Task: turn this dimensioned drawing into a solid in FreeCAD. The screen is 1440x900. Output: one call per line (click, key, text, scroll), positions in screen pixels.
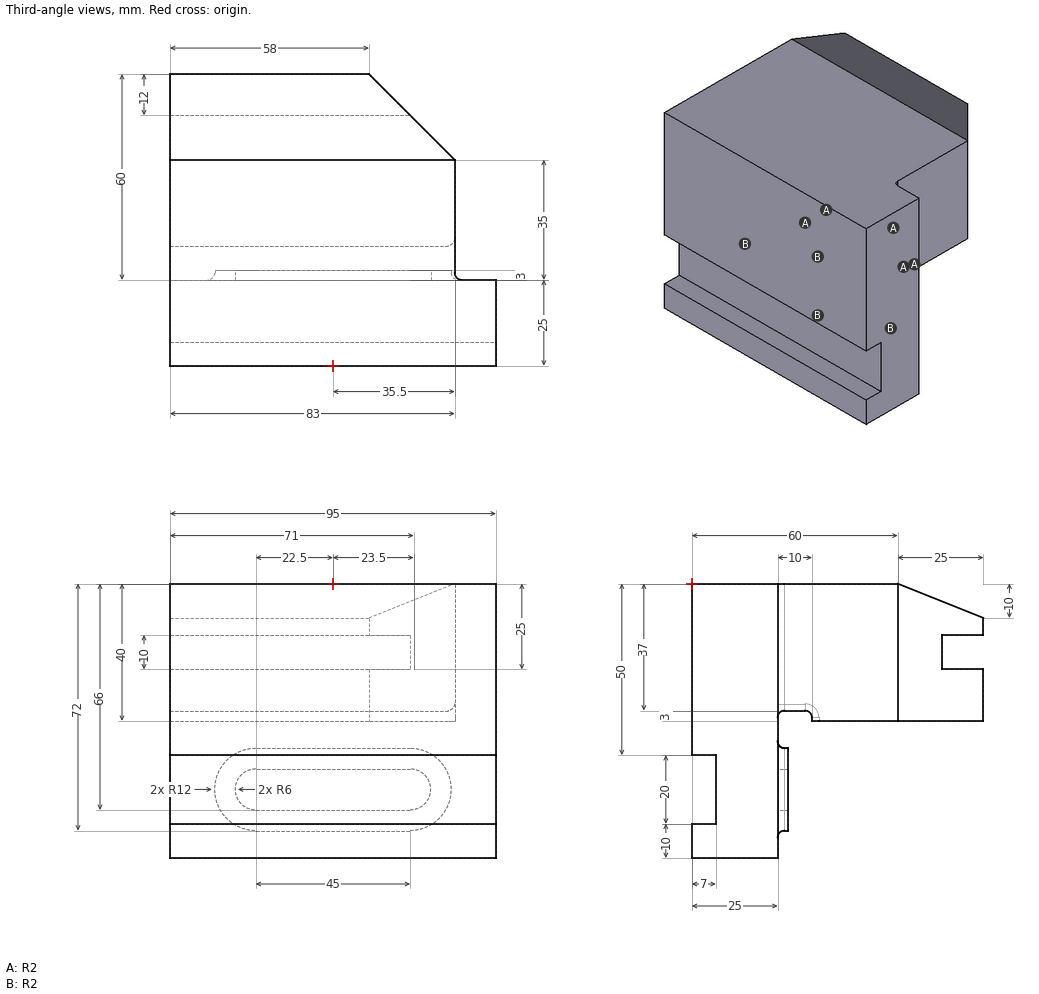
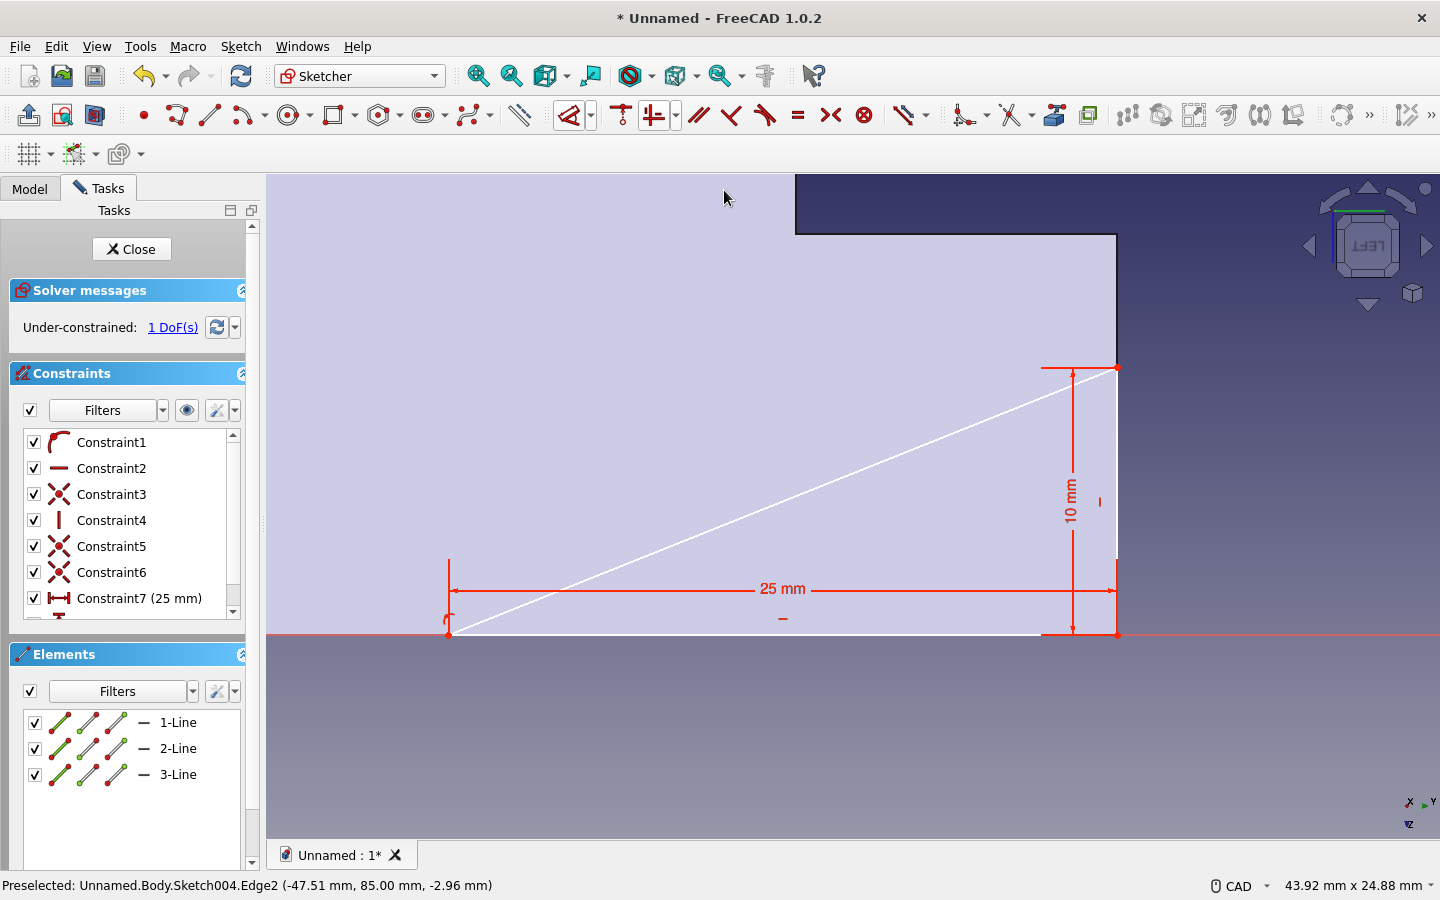
click(449, 635)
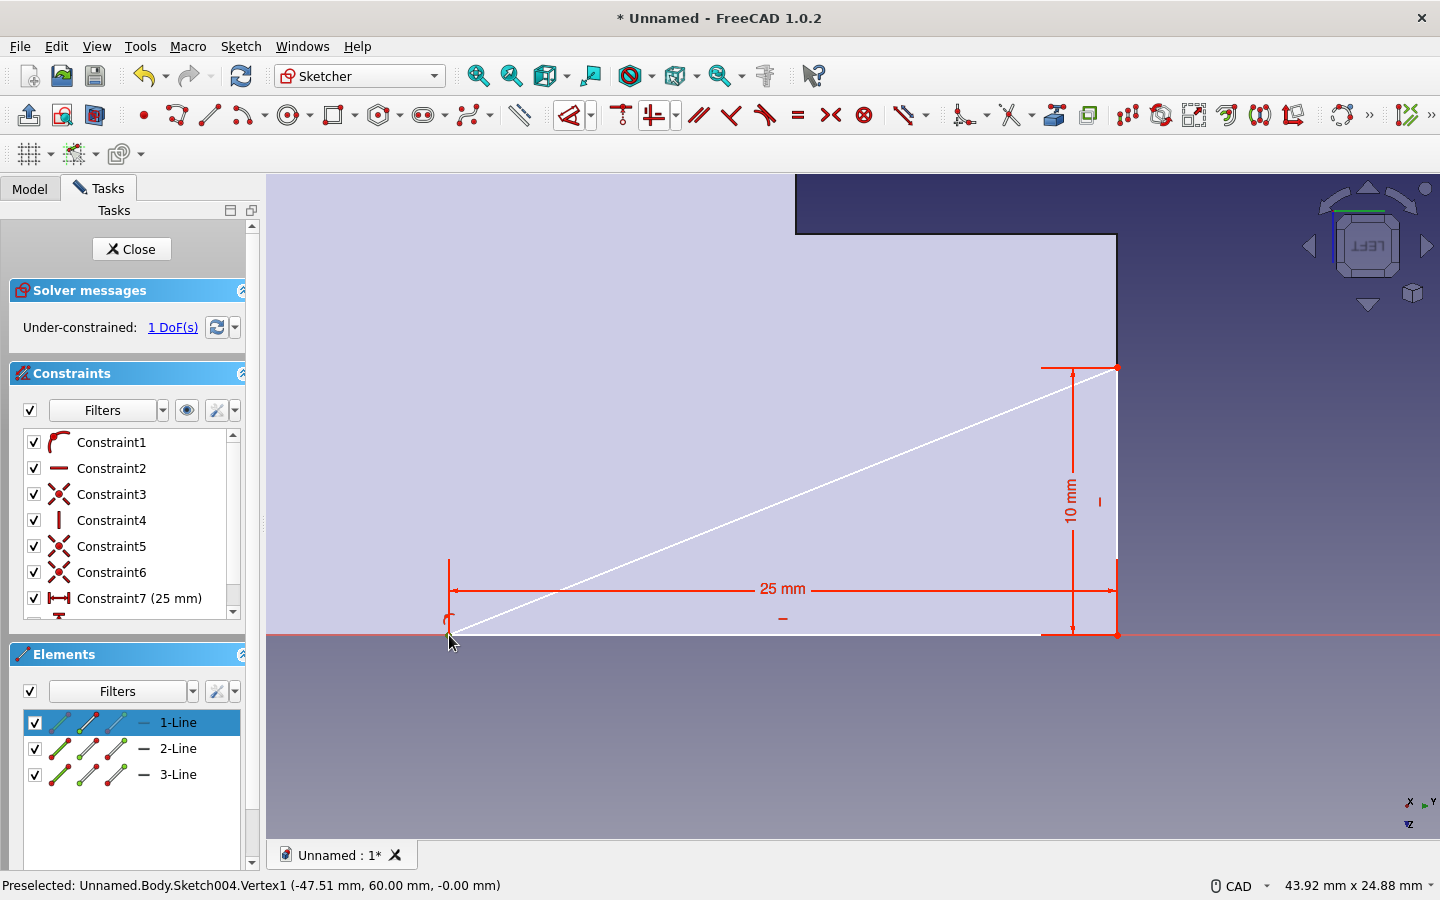
click(590, 116)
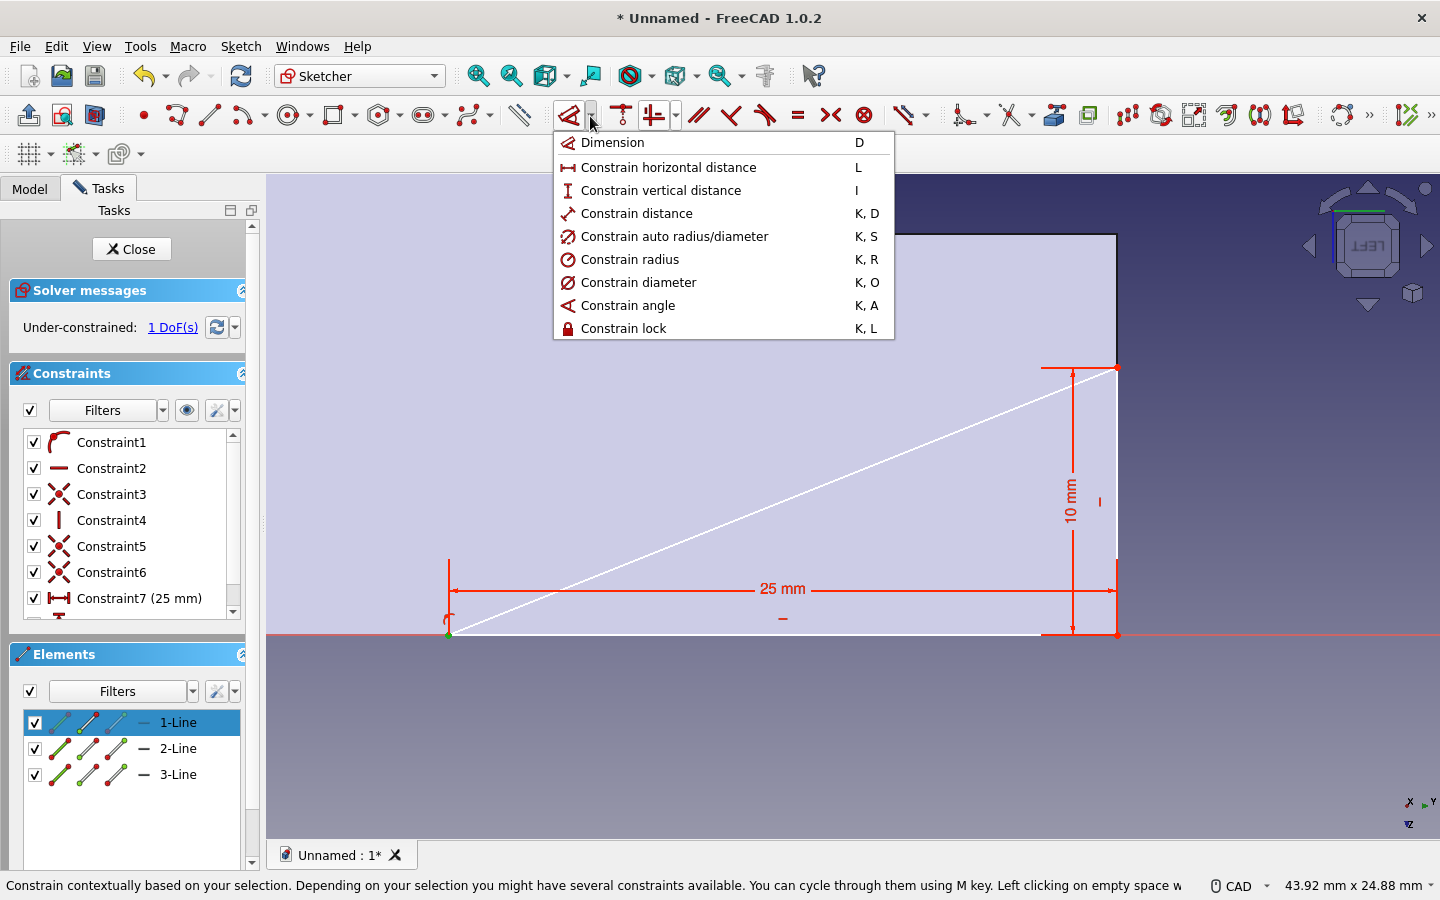
click(724, 168)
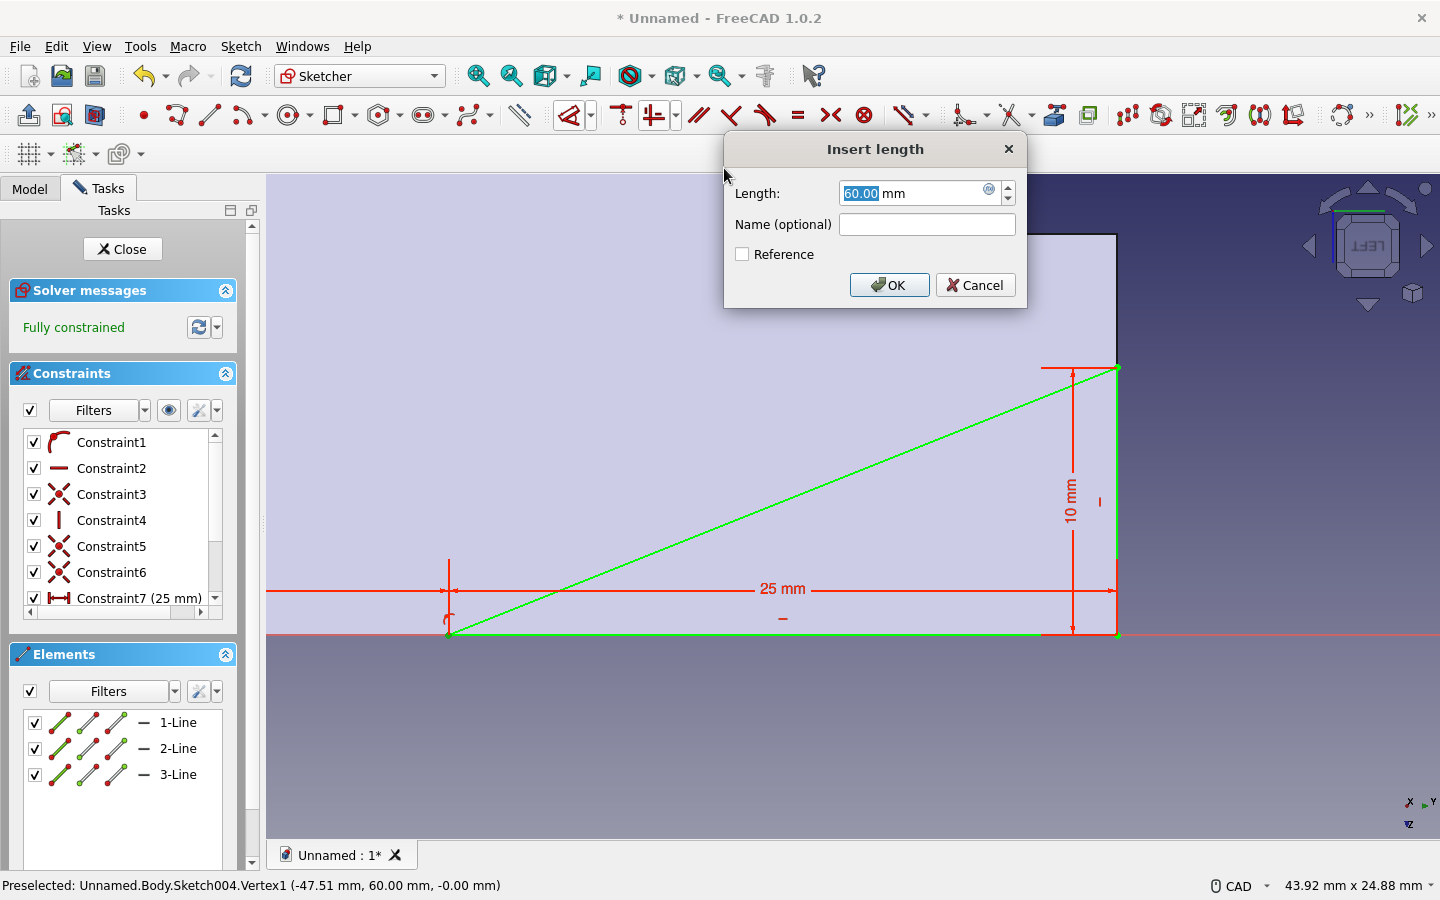
text(60)
key(Return)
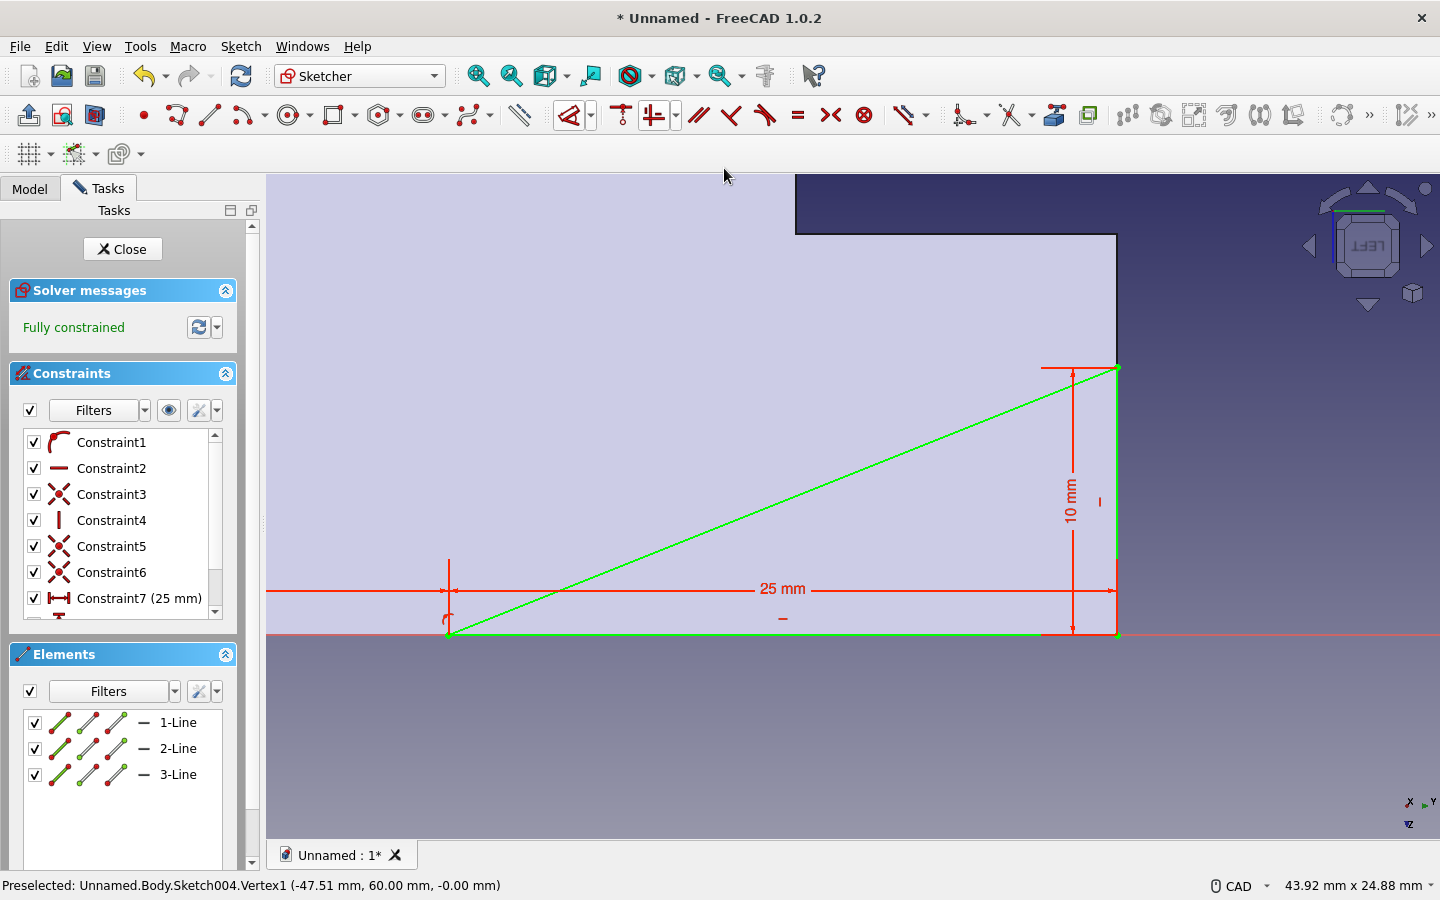
click(123, 249)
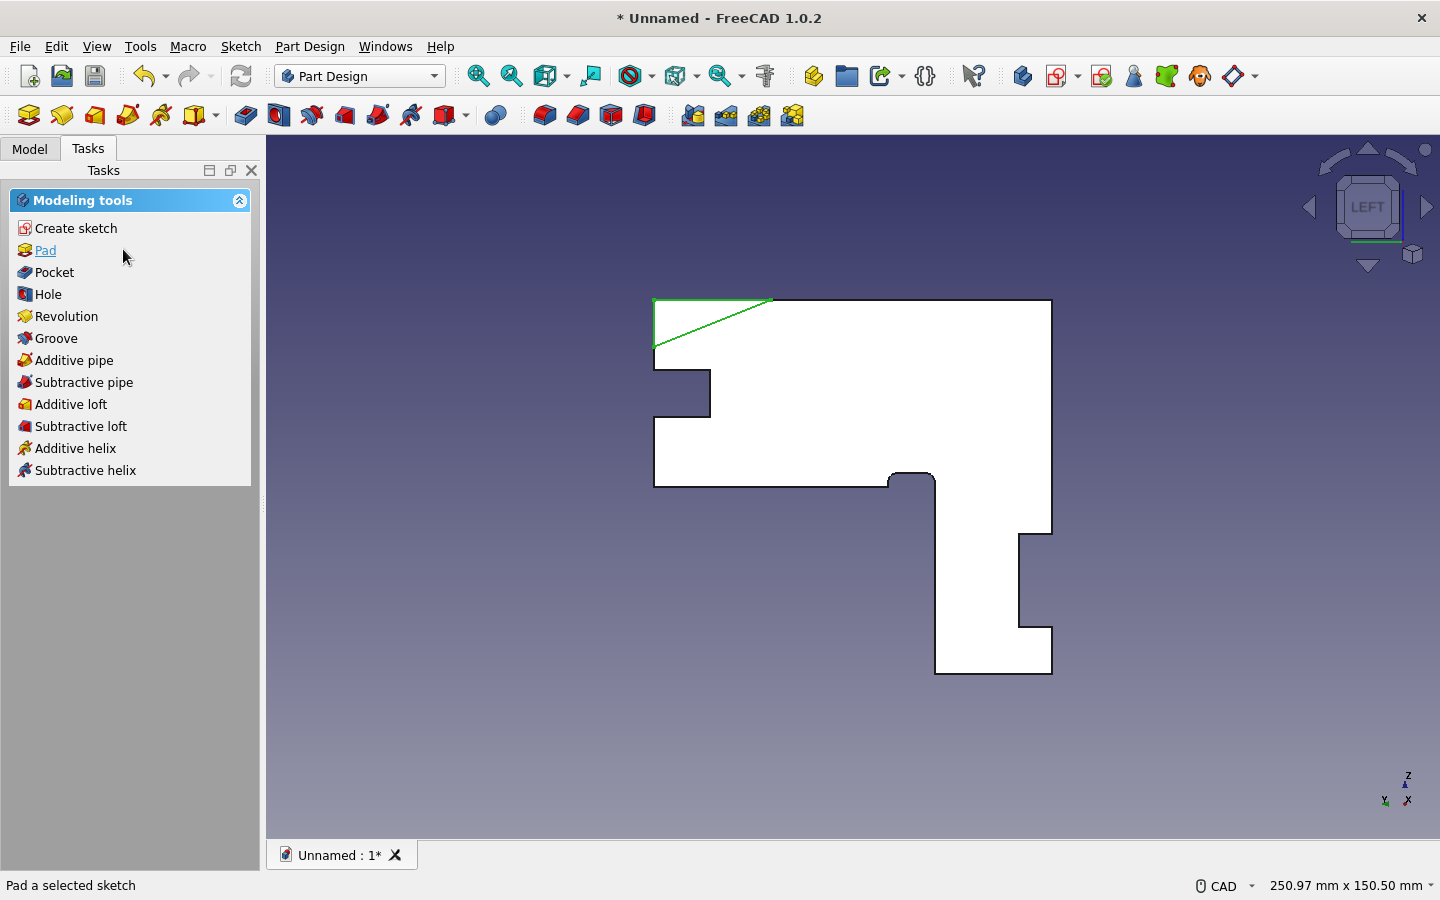
click(246, 116)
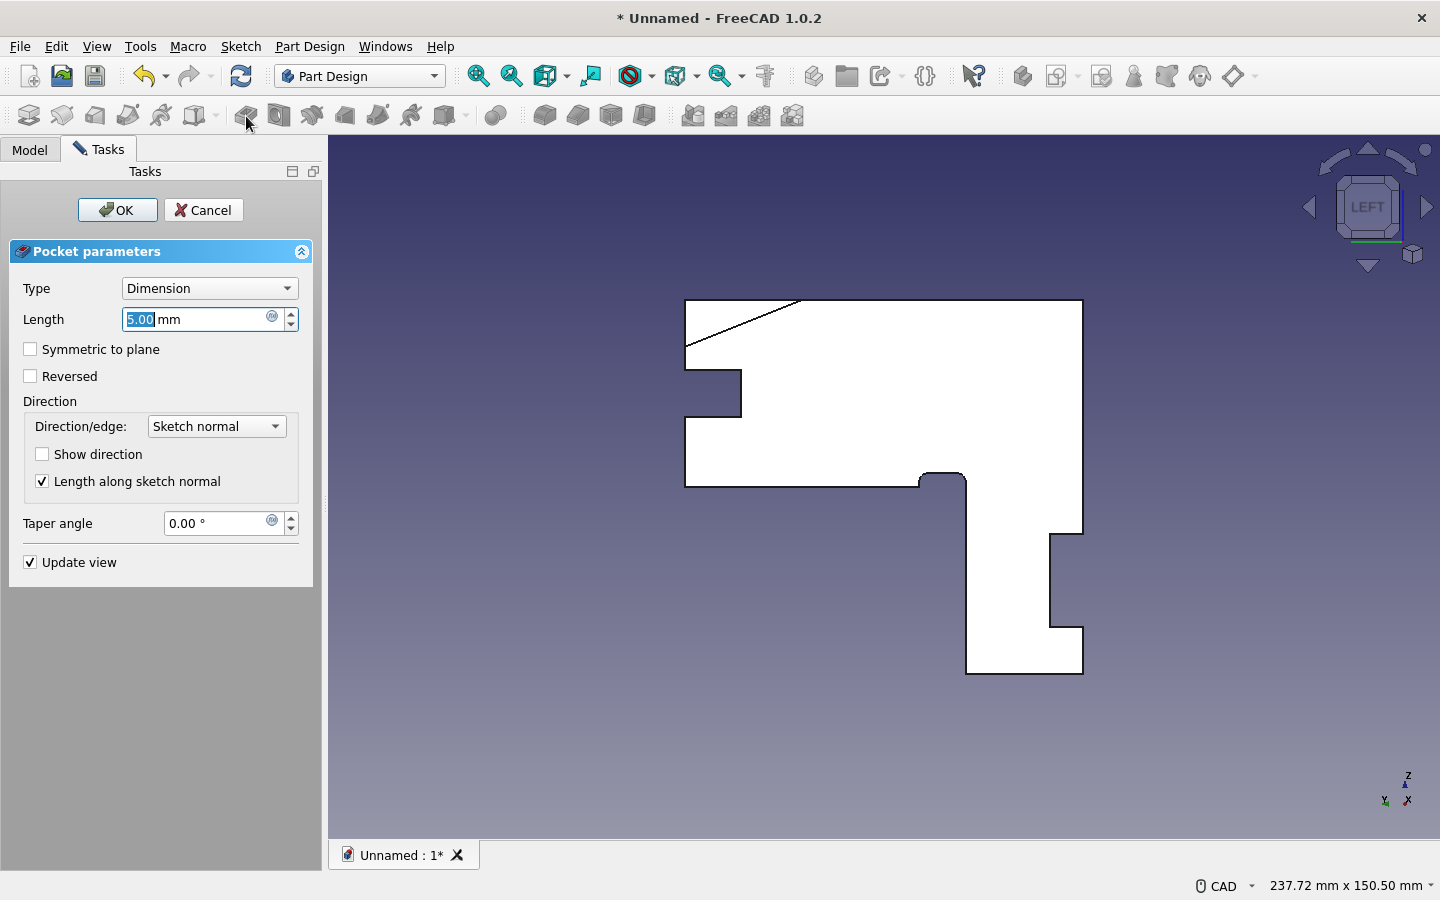
click(210, 288)